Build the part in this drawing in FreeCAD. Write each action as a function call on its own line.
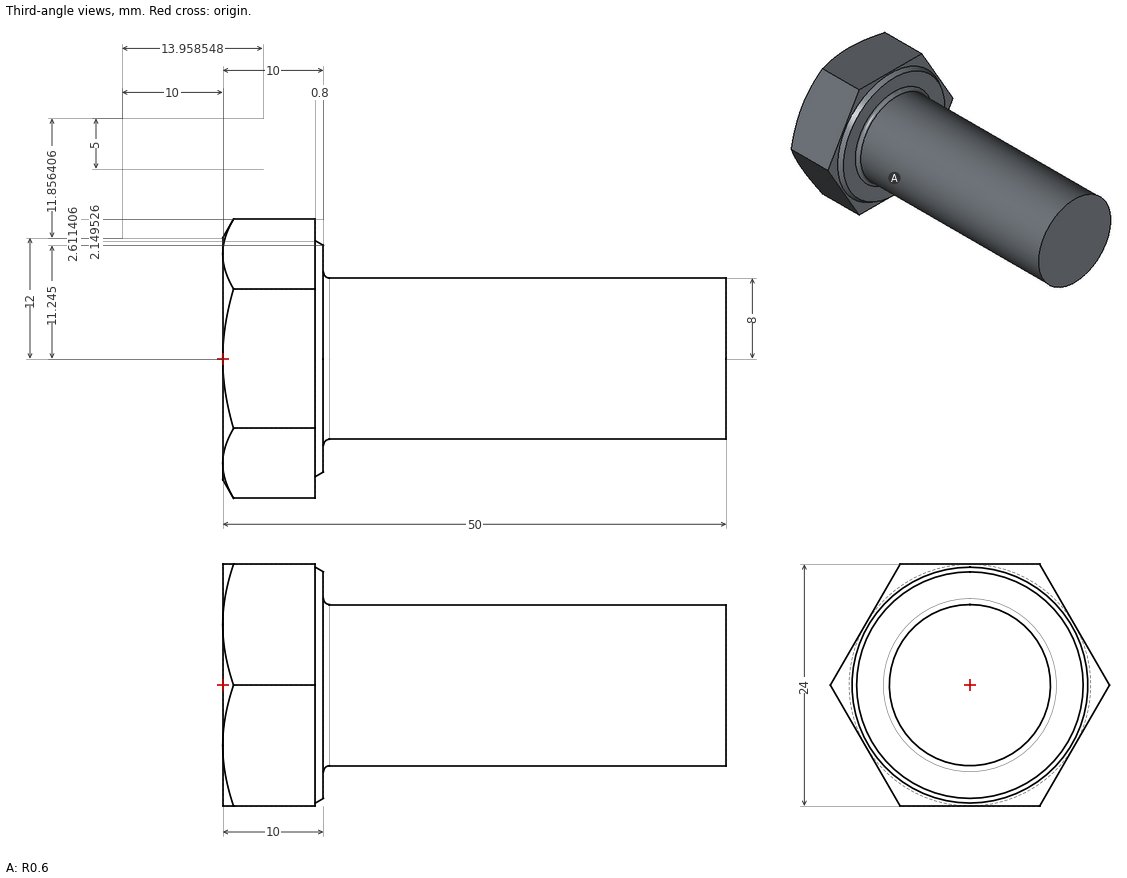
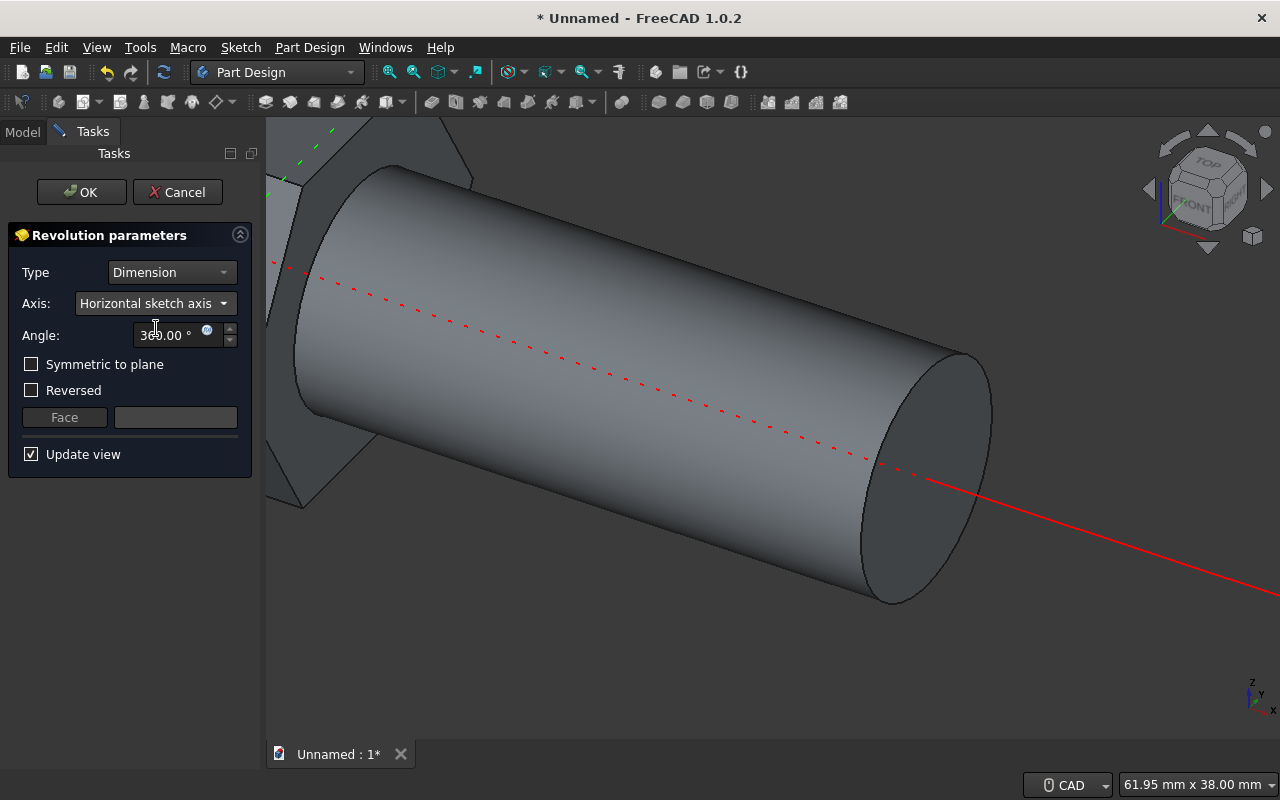
click(82, 192)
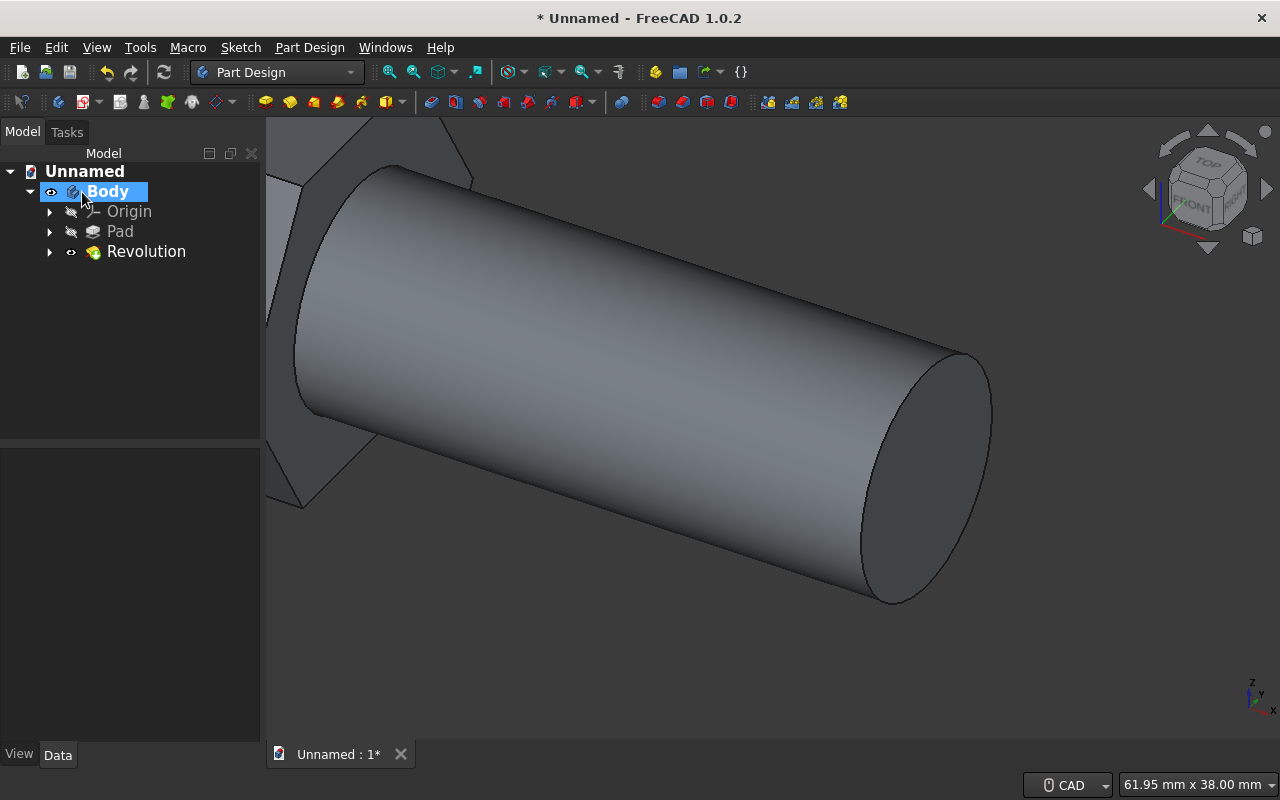
click(390, 72)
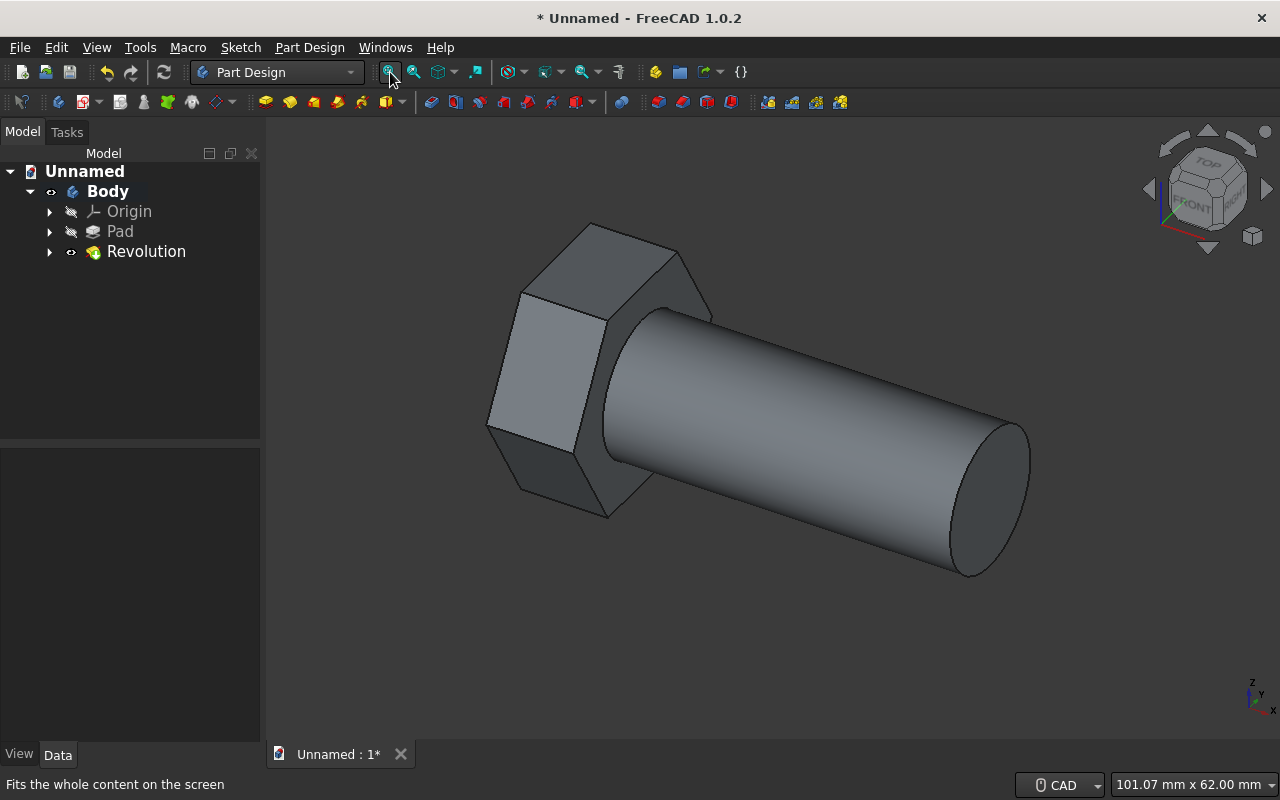
click(84, 102)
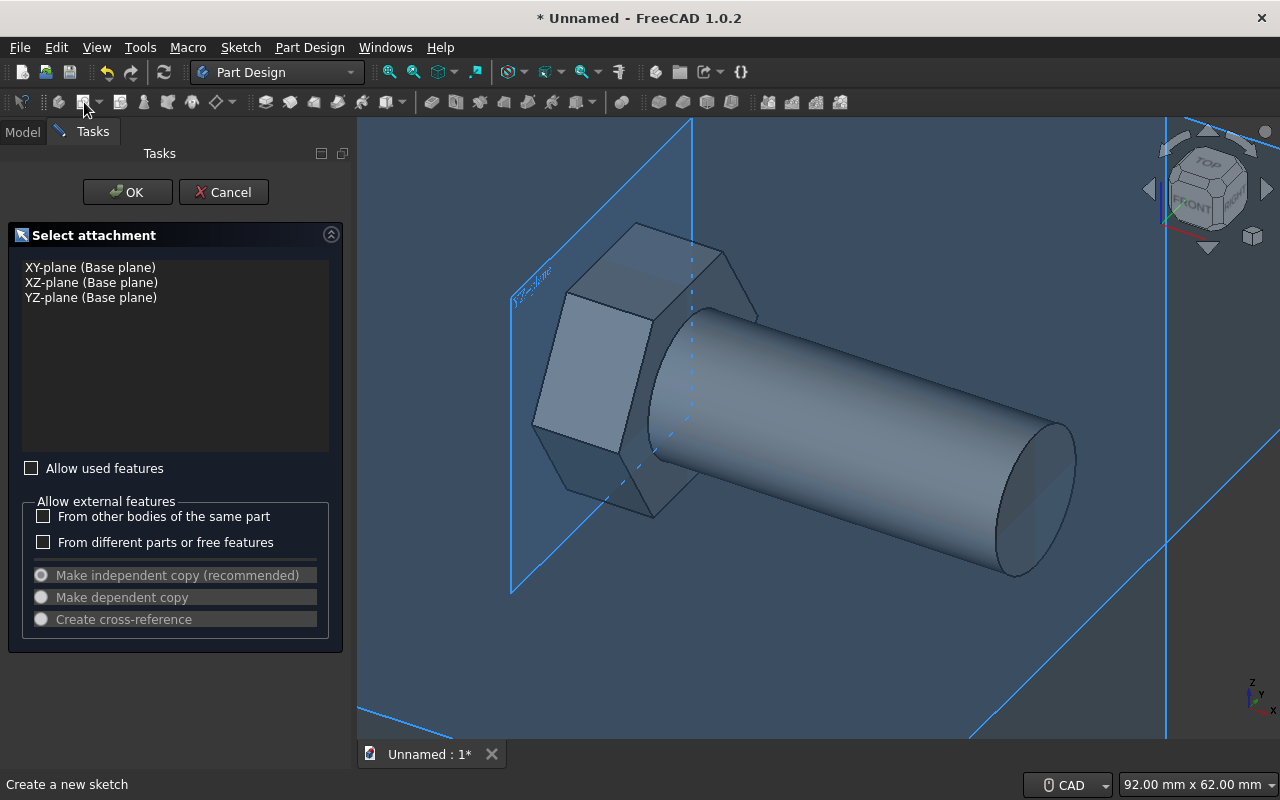
click(82, 268)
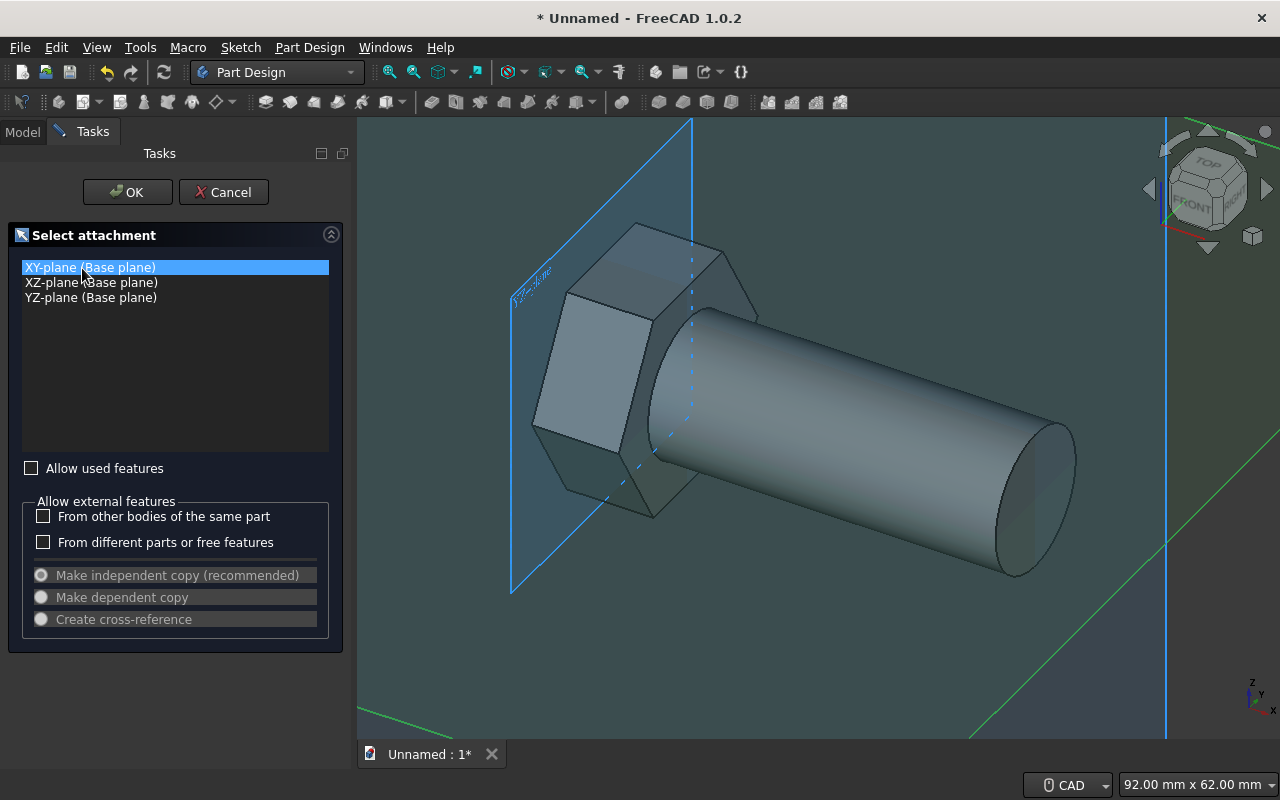
click(128, 192)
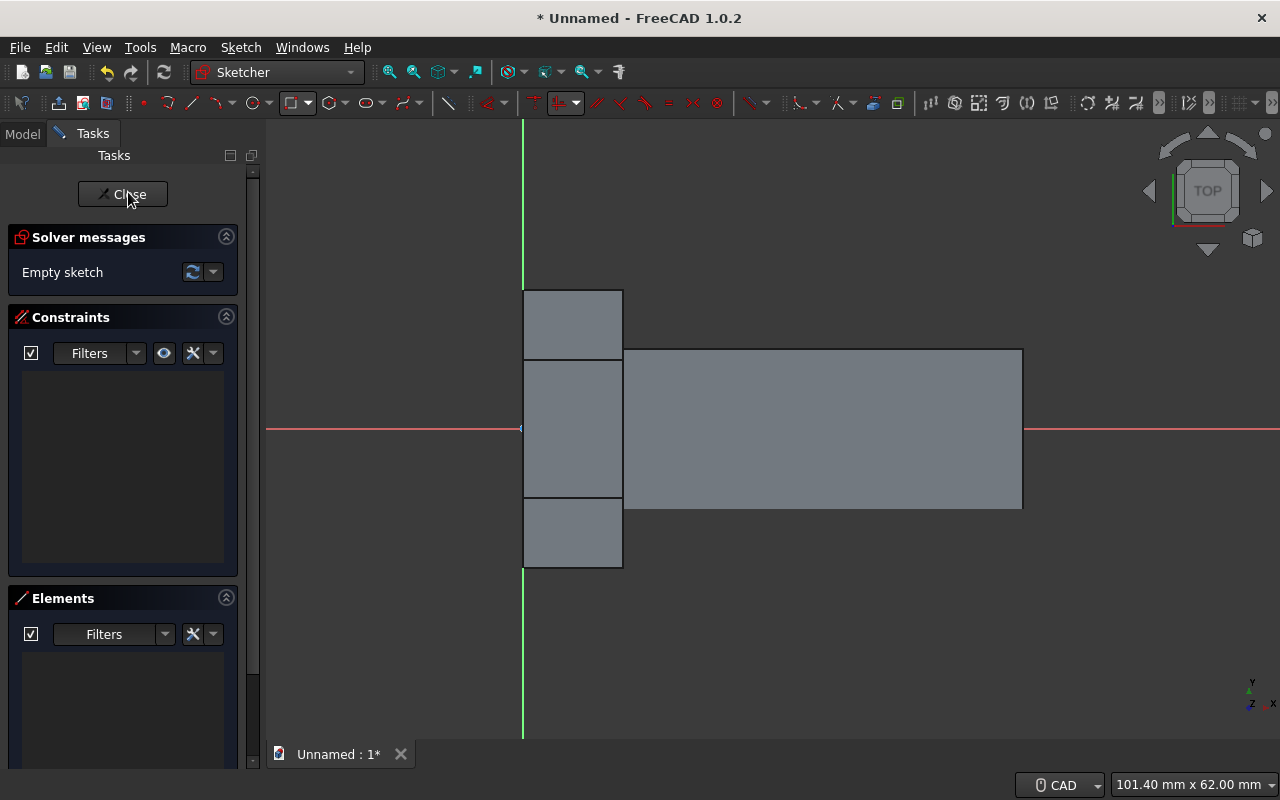
click(108, 104)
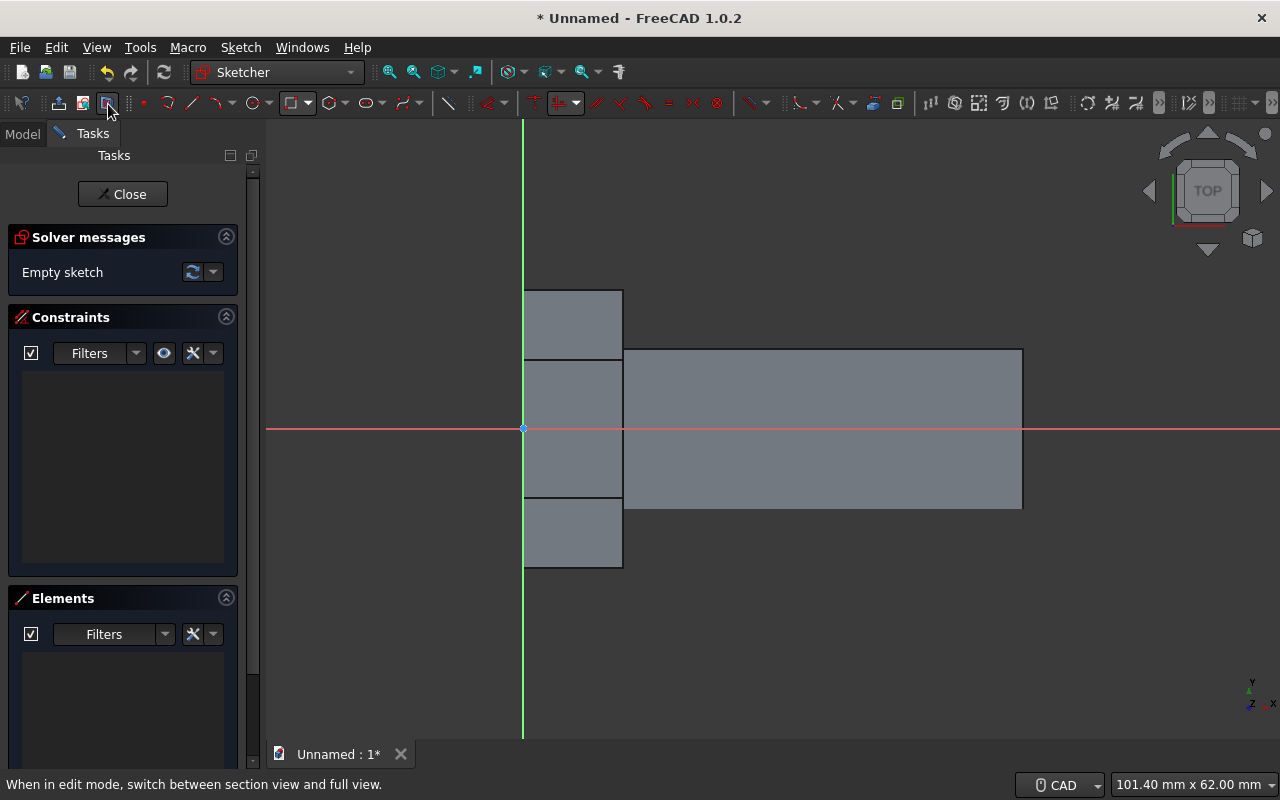
scroll(294, 165, up, 3)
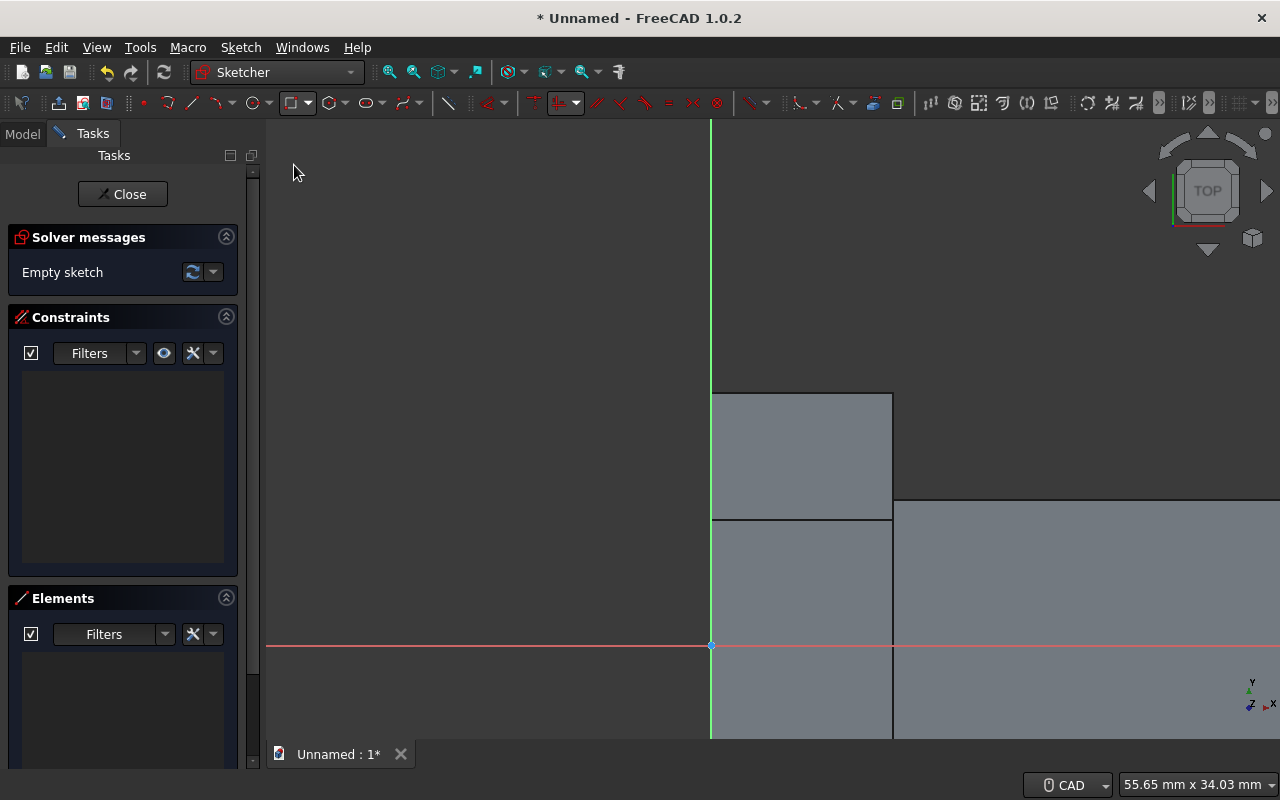
click(168, 104)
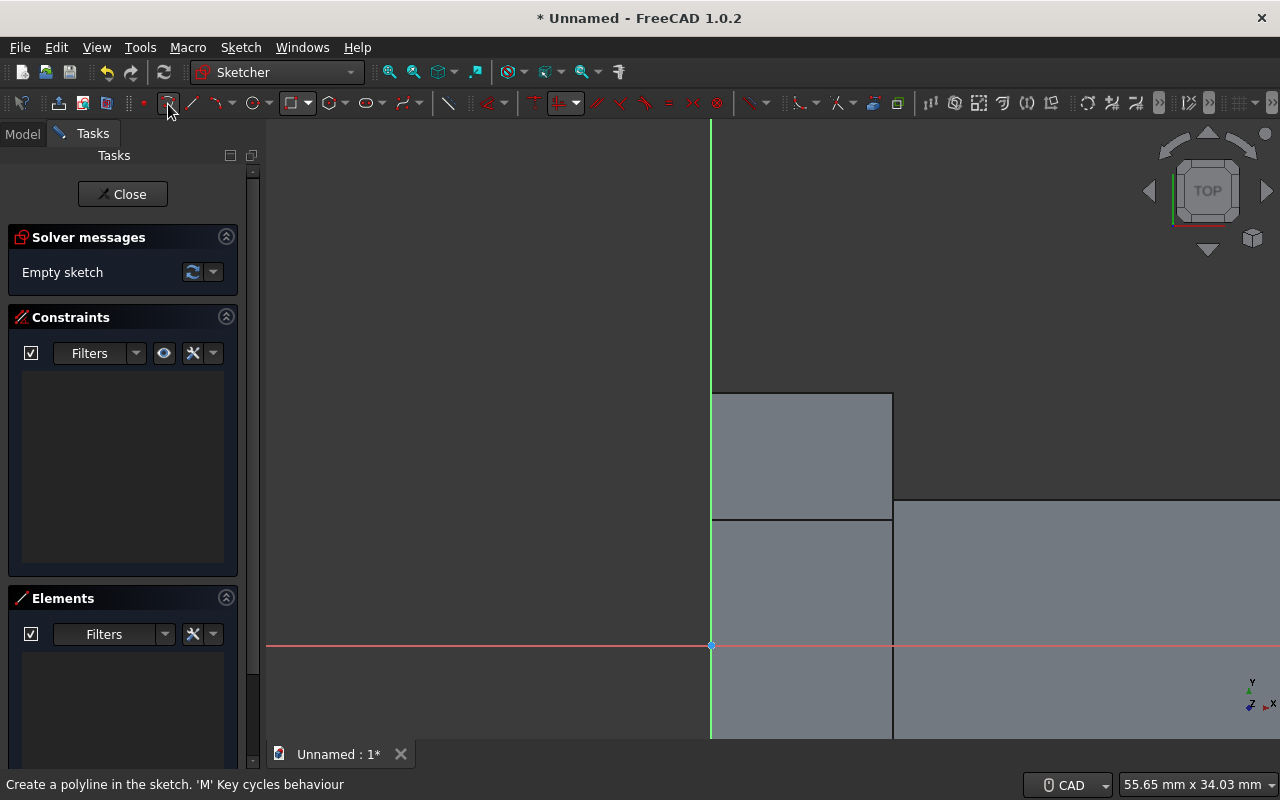
click(711, 427)
click(783, 302)
click(783, 211)
click(529, 211)
click(529, 427)
click(711, 428)
key(Escape)
key(Escape)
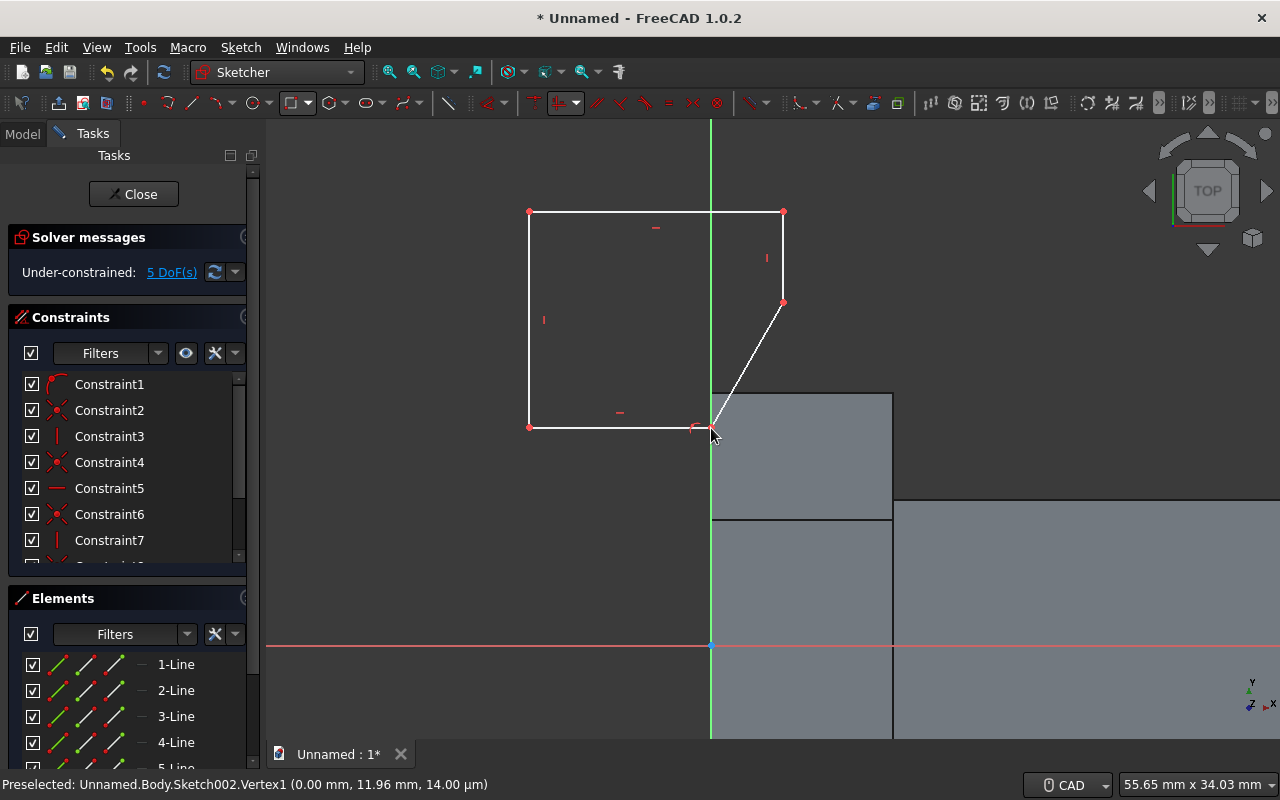
click(488, 104)